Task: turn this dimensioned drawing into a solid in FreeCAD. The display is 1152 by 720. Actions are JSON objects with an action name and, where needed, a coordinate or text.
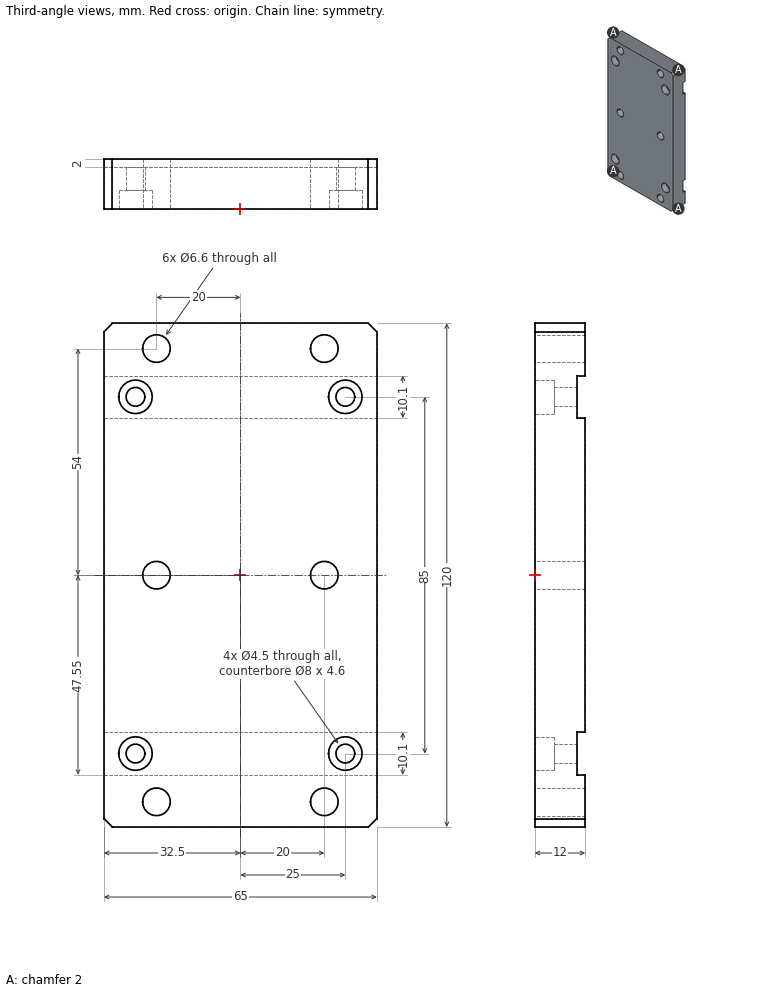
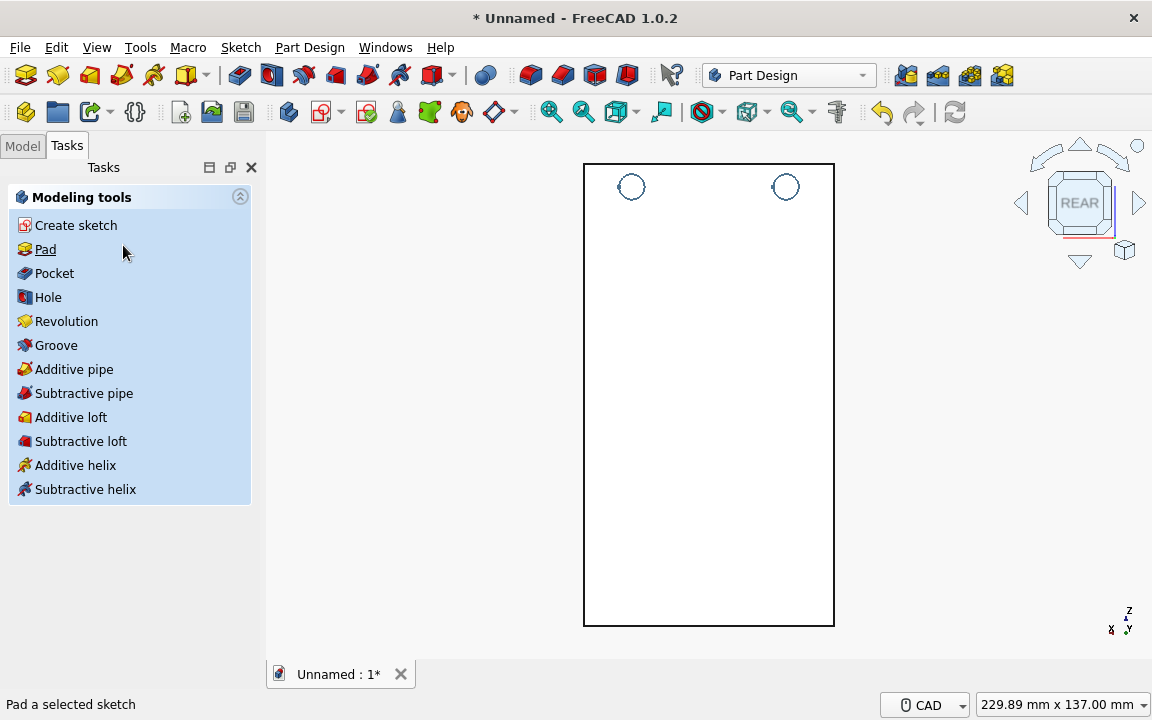
{"action": "left_click", "coordinate": [272, 76]}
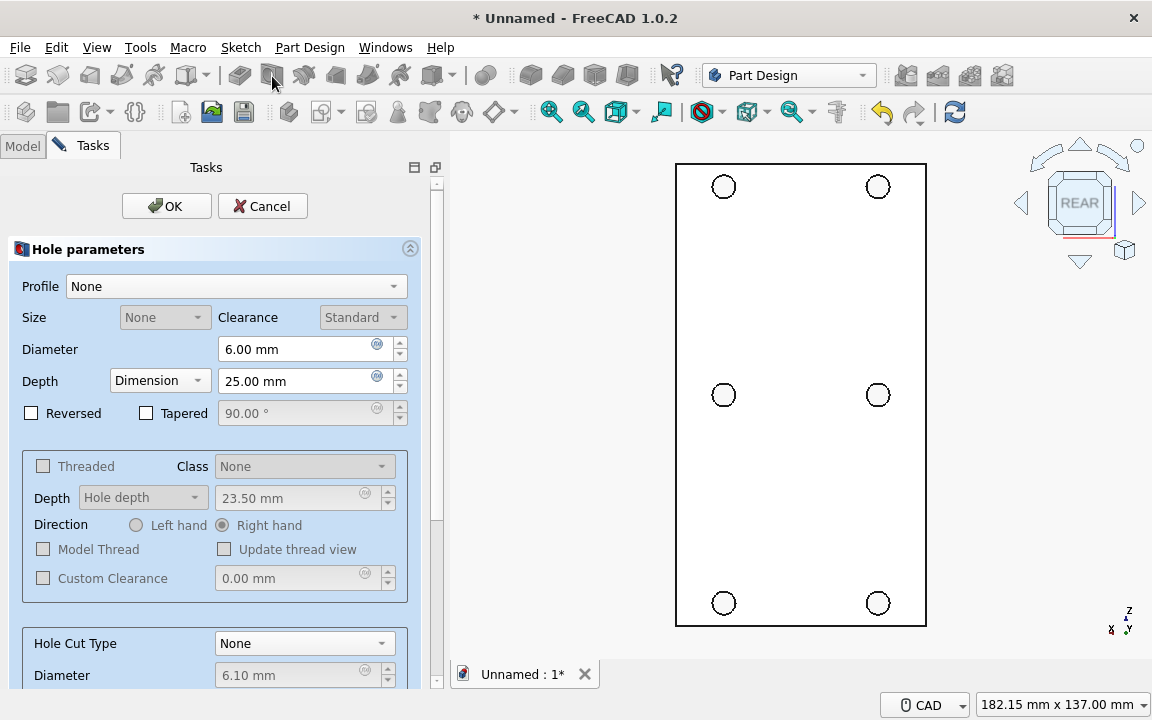
{"action": "triple_click", "coordinate": [305, 349]}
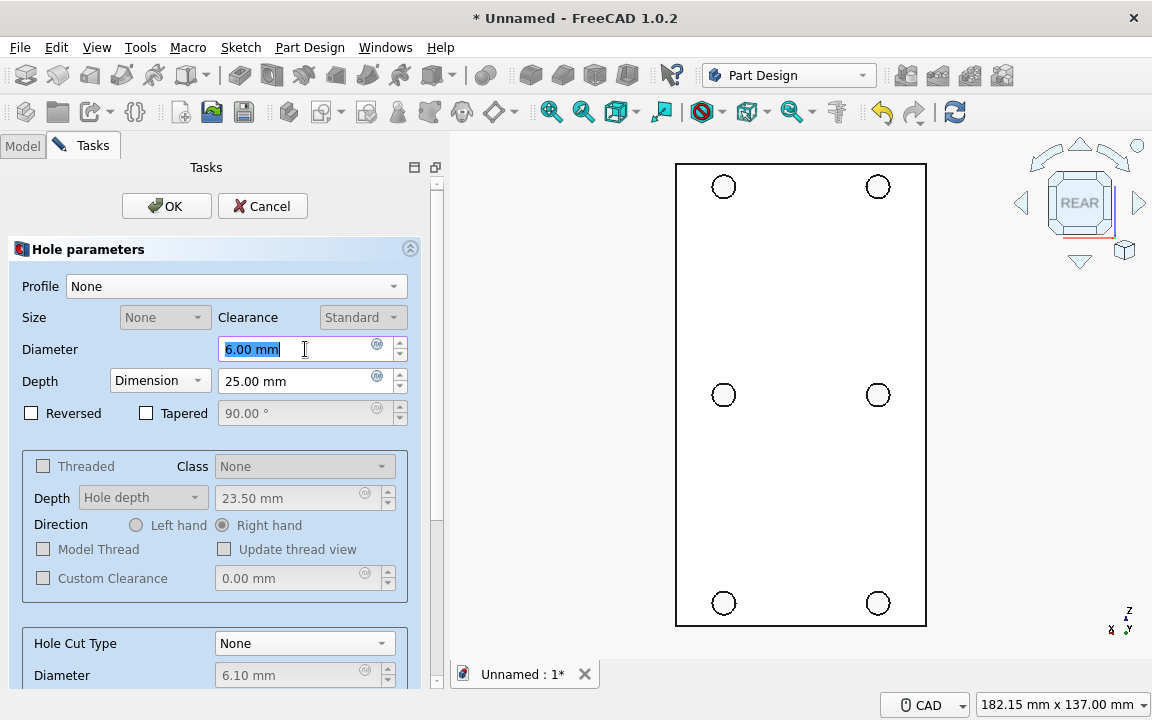
{"action": "type", "text": "6.6"}
{"action": "key", "text": "Tab"}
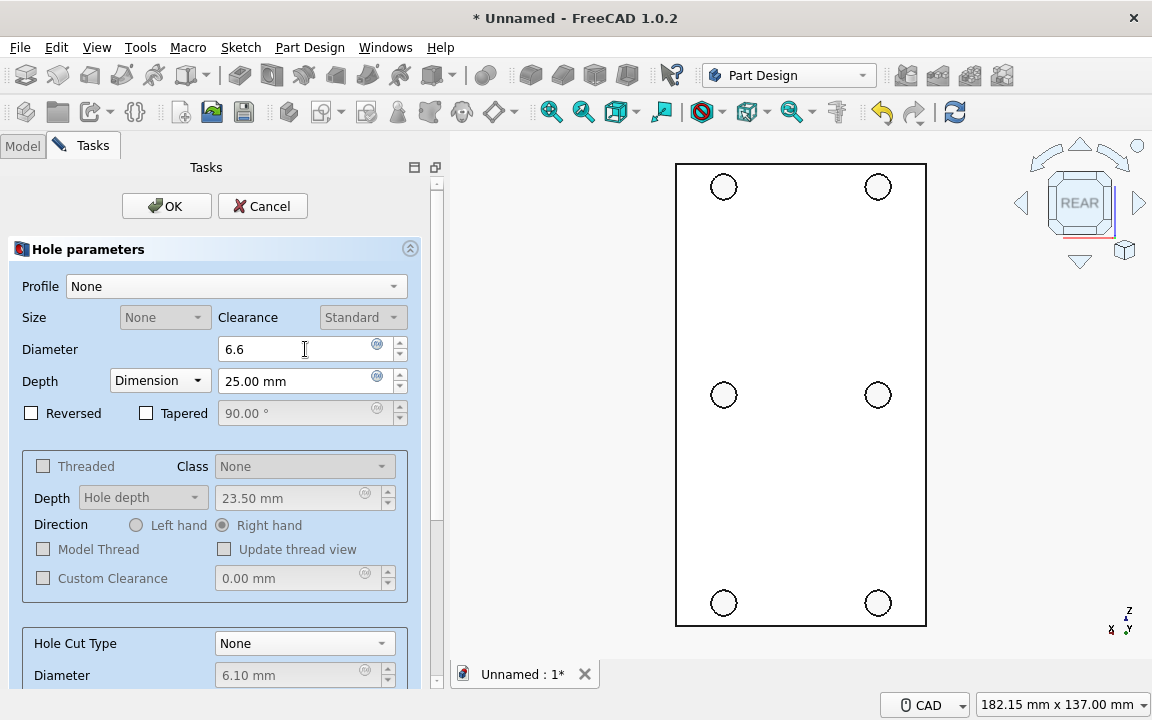
{"action": "left_click", "coordinate": [161, 380]}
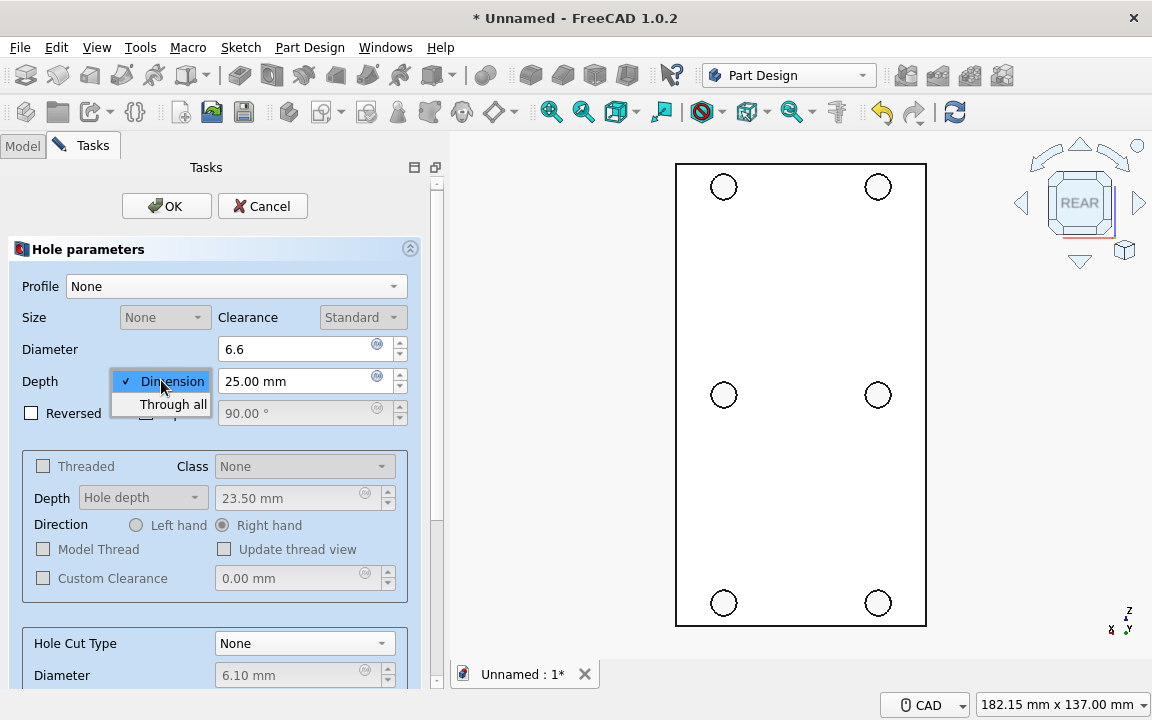
{"action": "left_click", "coordinate": [160, 404]}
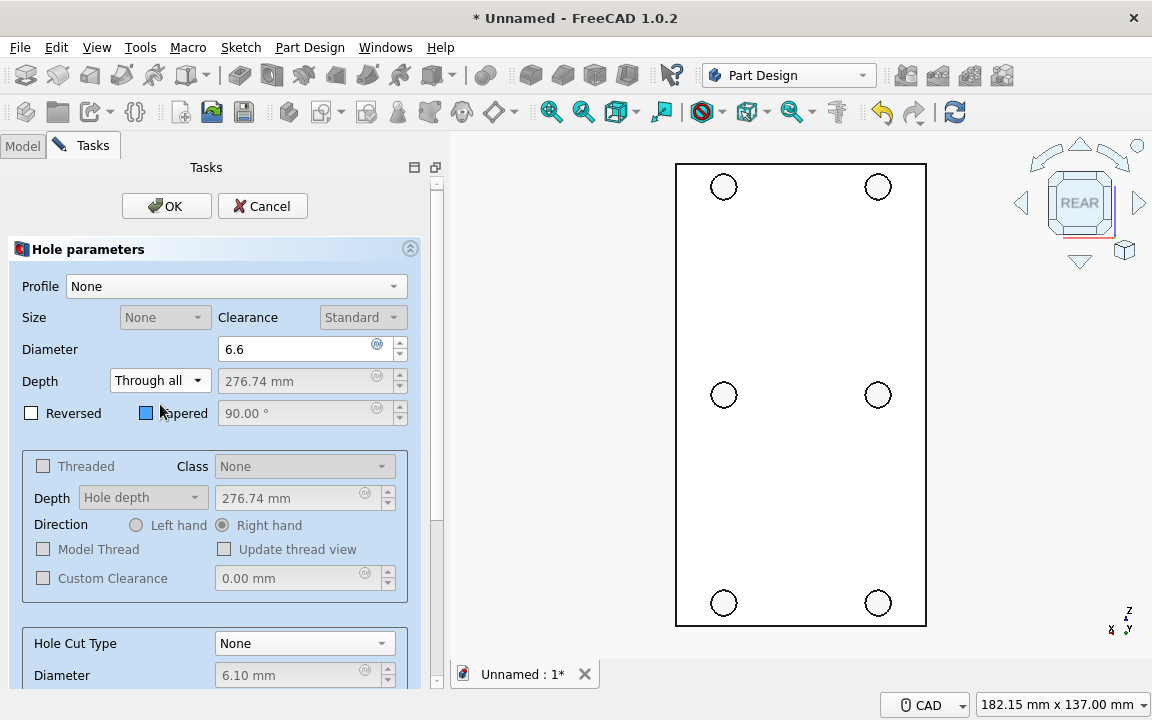
{"action": "left_click", "coordinate": [167, 206]}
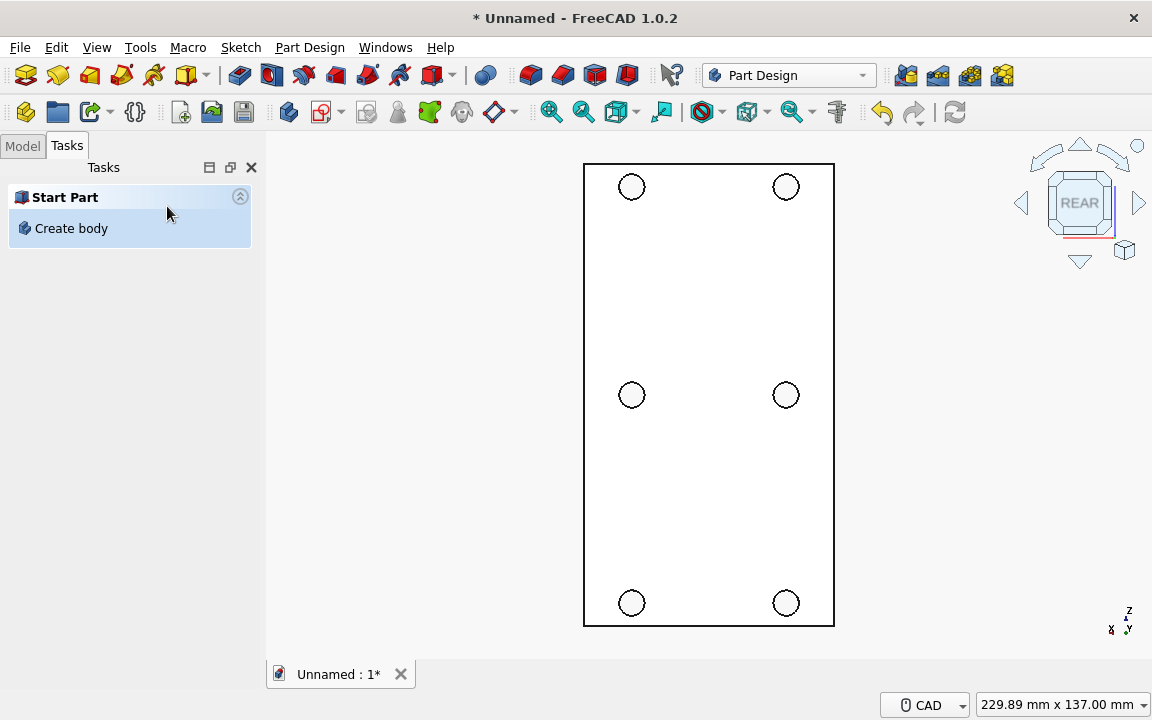
{"action": "left_click", "coordinate": [709, 526]}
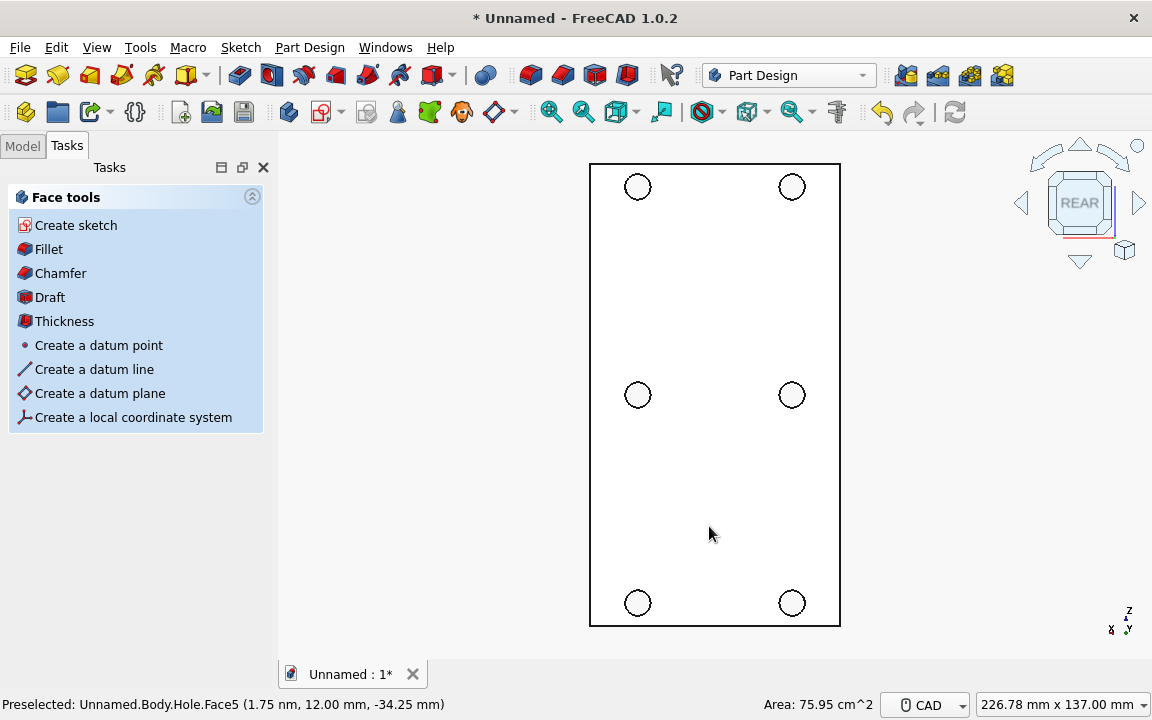
{"action": "left_click", "coordinate": [322, 112]}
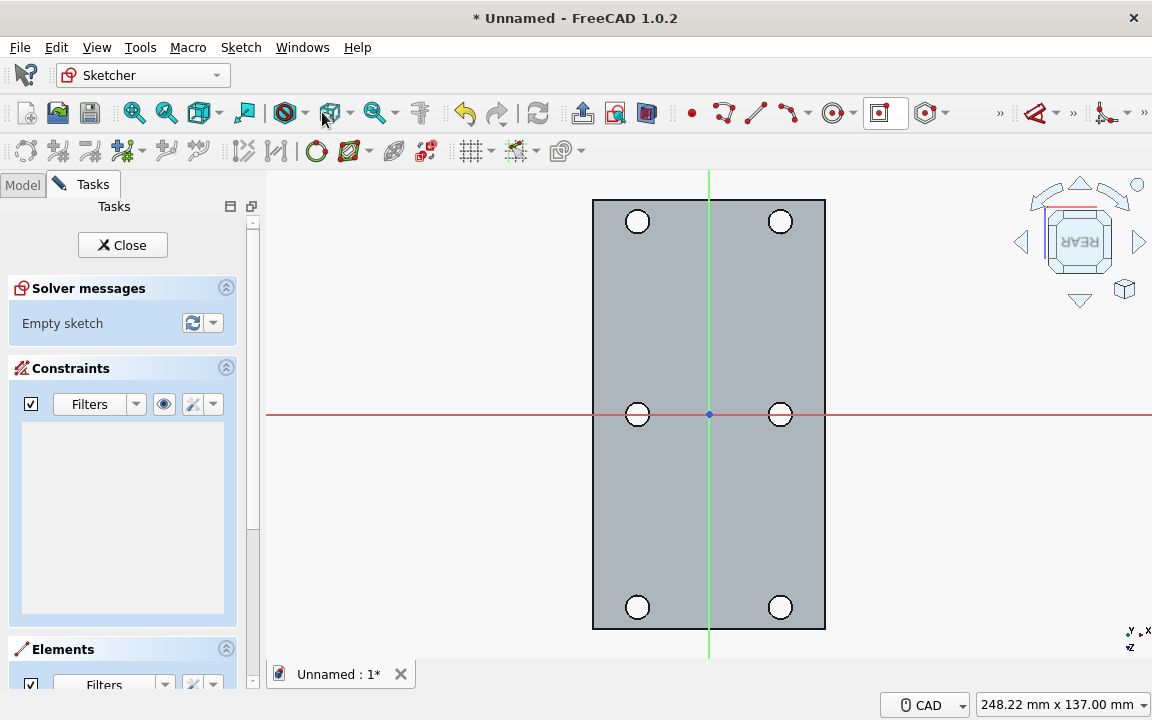
{"action": "left_click", "coordinate": [902, 114]}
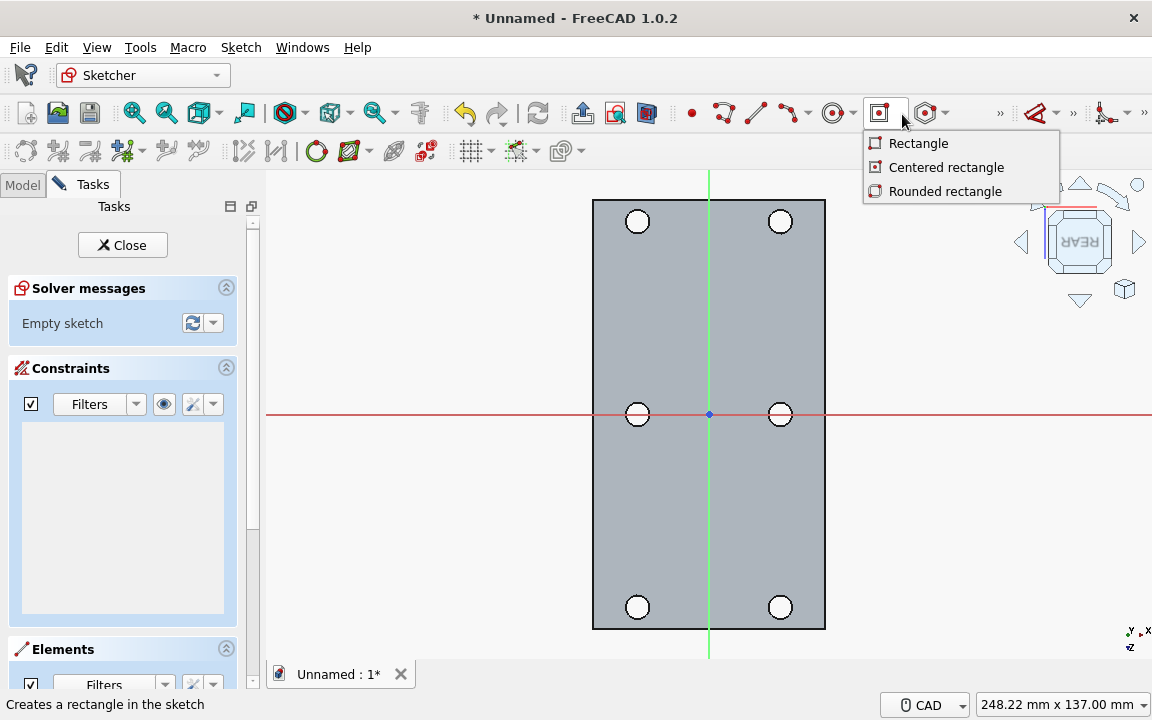
{"action": "left_click", "coordinate": [962, 143]}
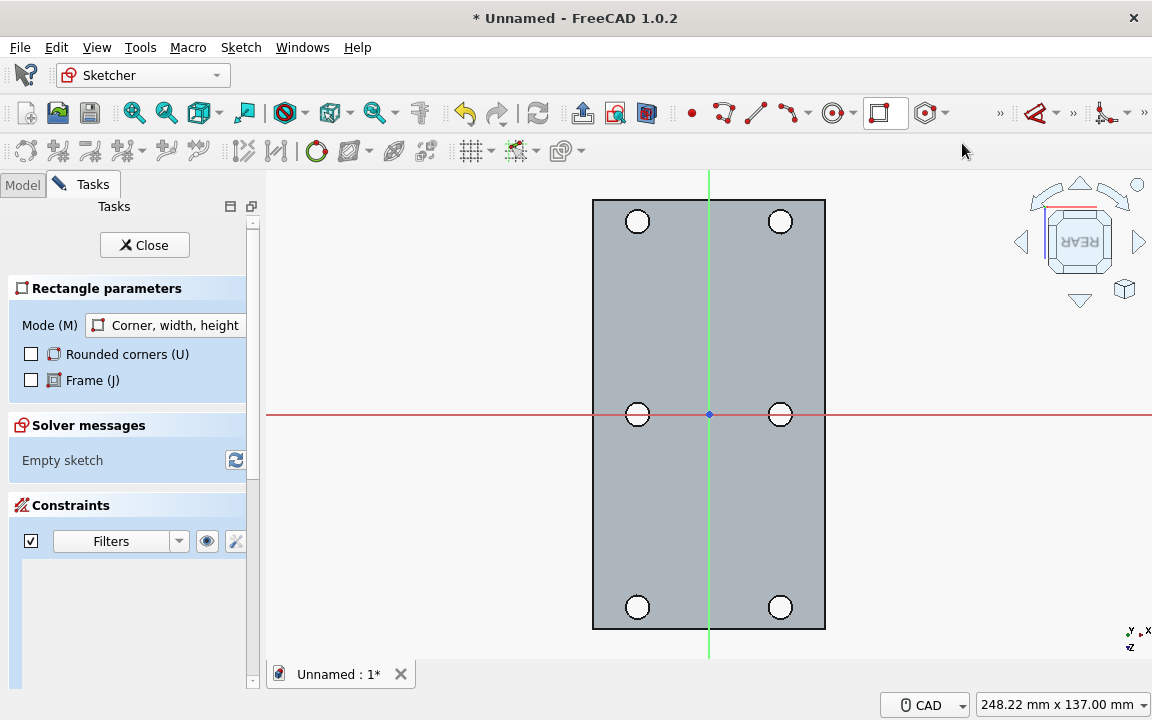
{"action": "left_click", "coordinate": [593, 245]}
{"action": "mouse_move", "coordinate": [825, 281]}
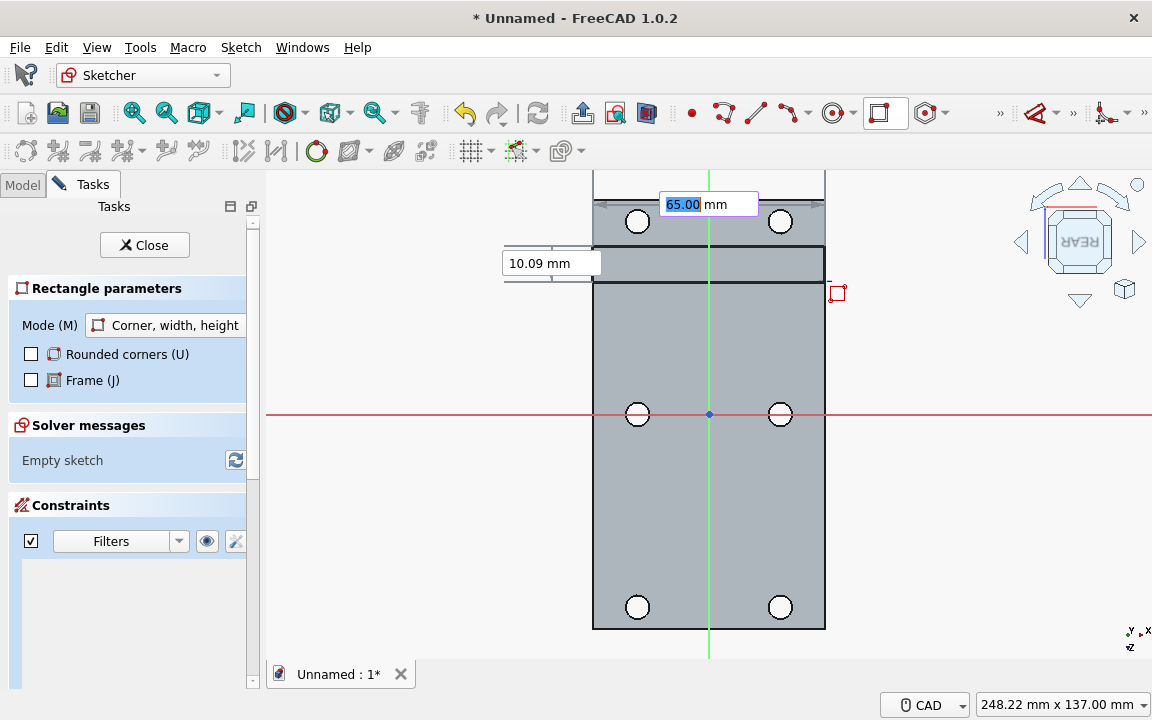
{"action": "type", "text": "65"}
{"action": "key", "text": "Tab"}
{"action": "type", "text": "10.1"}
{"action": "key", "text": "Return"}